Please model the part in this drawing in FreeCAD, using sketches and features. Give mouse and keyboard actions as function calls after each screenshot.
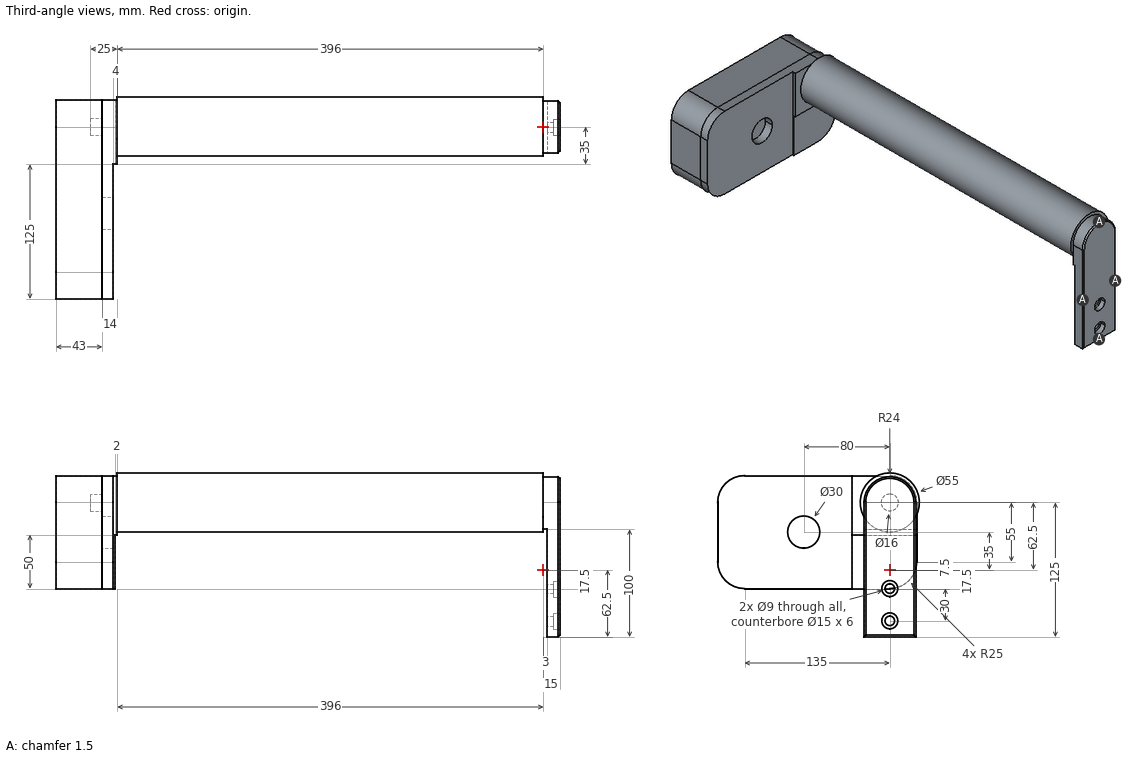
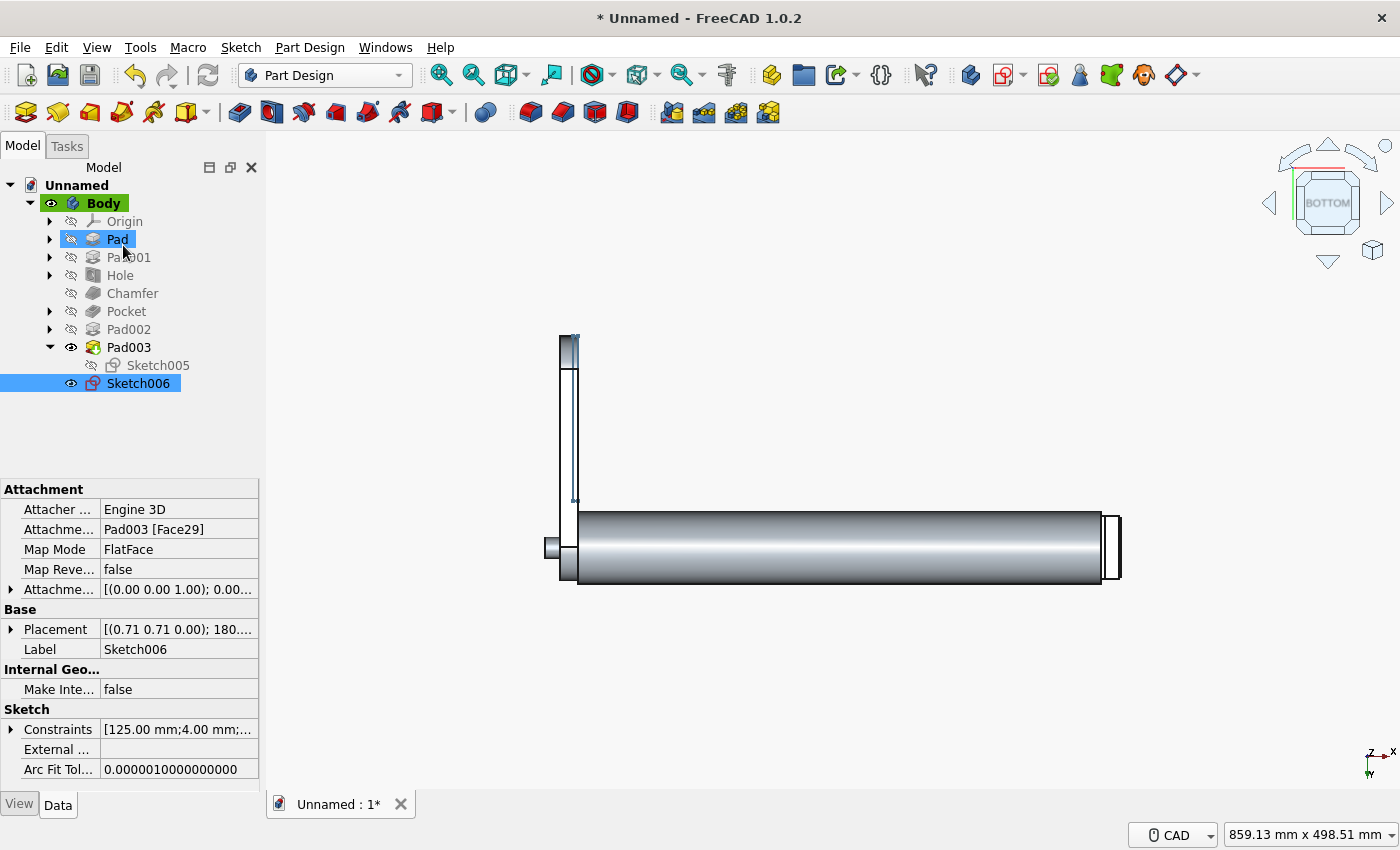
click(240, 112)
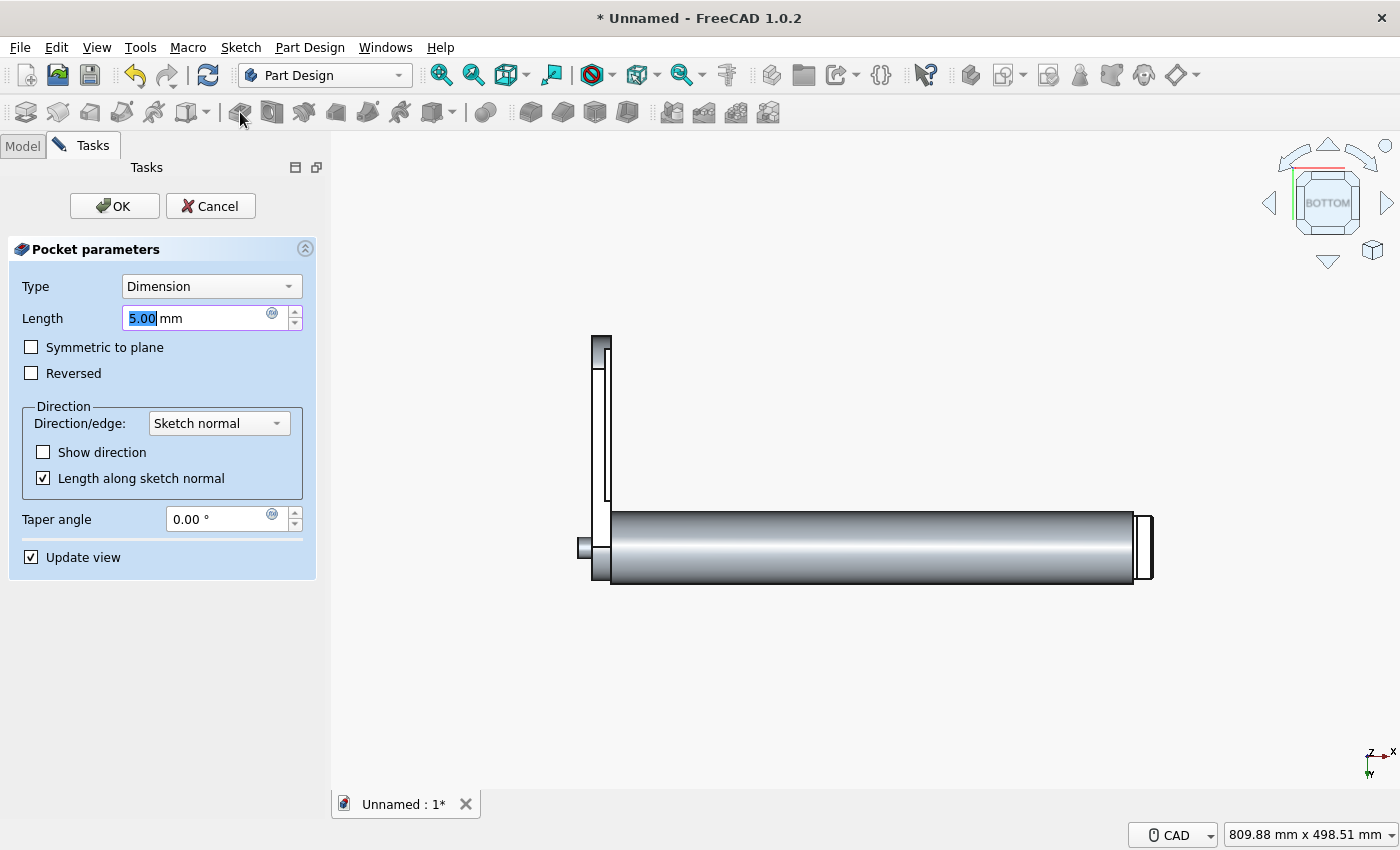
click(212, 286)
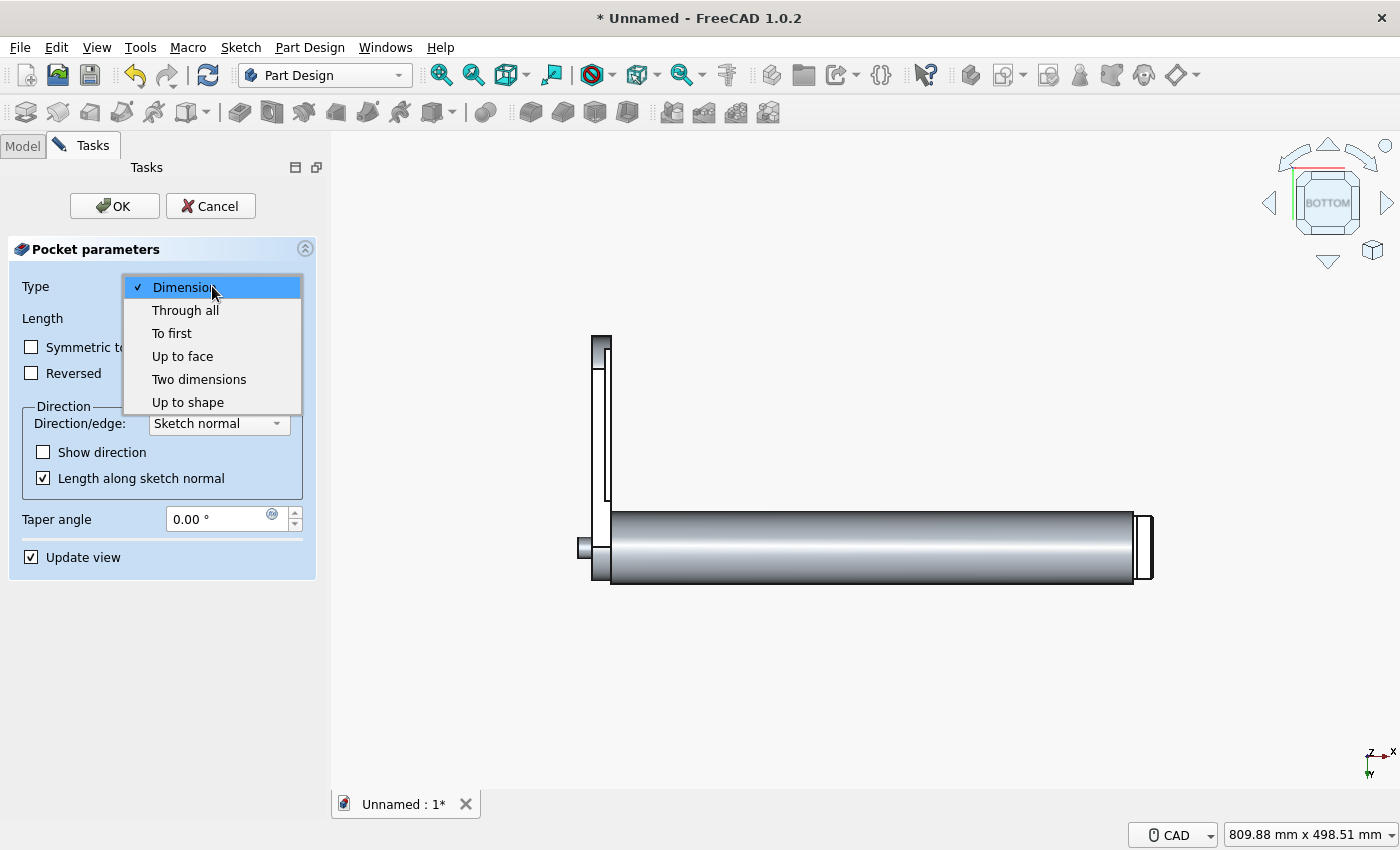
click(212, 310)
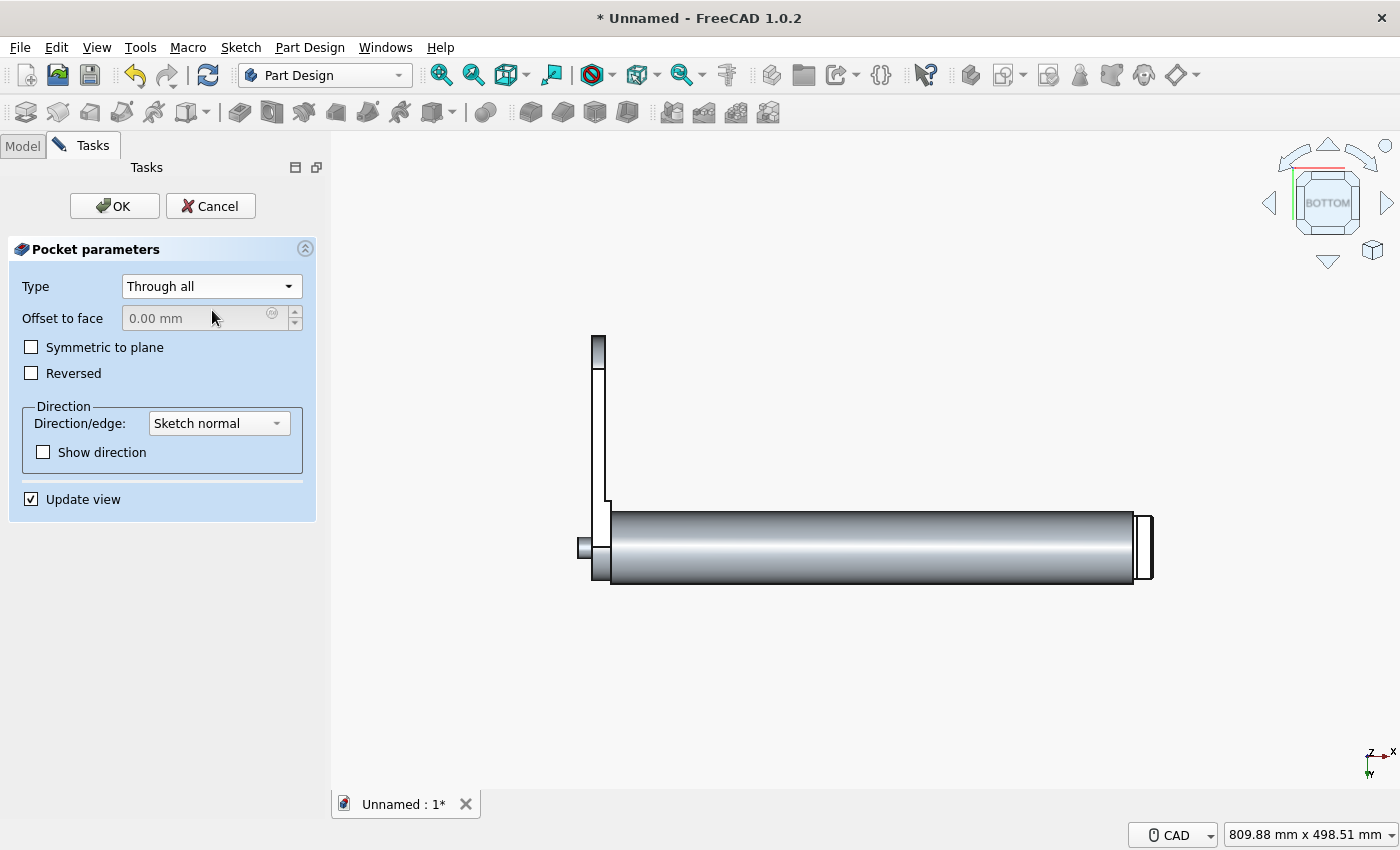
click(115, 206)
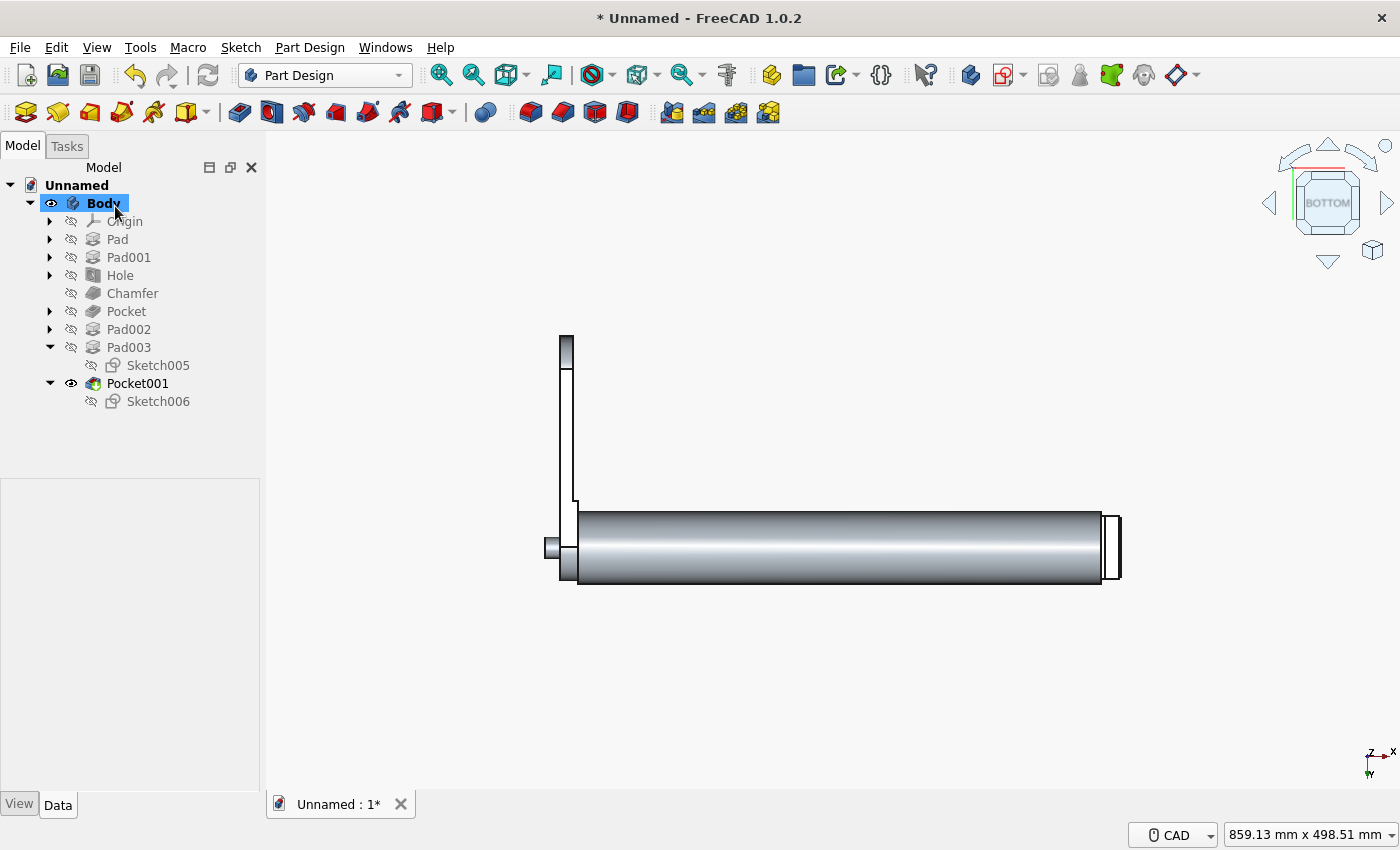
key(0)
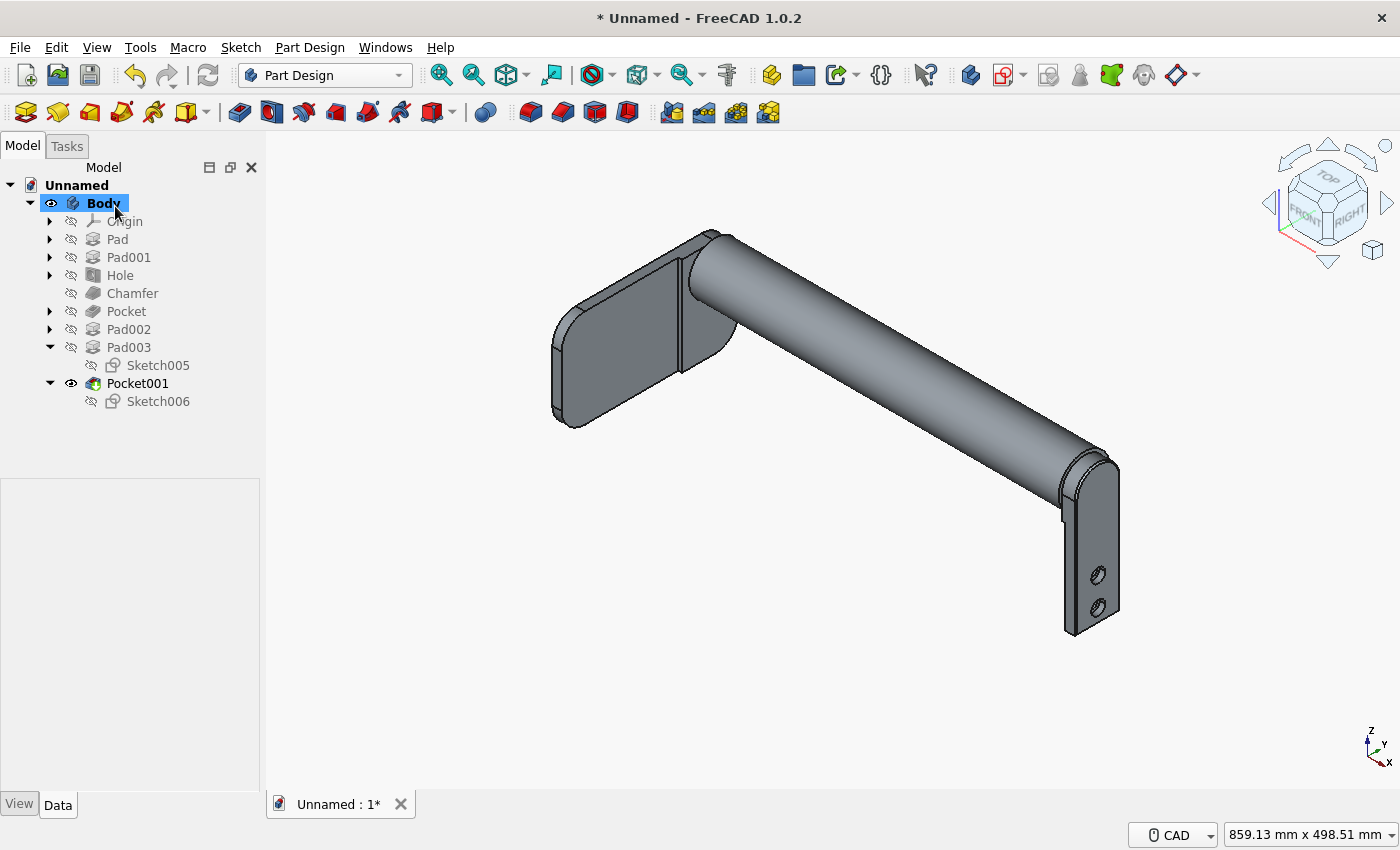
click(620, 347)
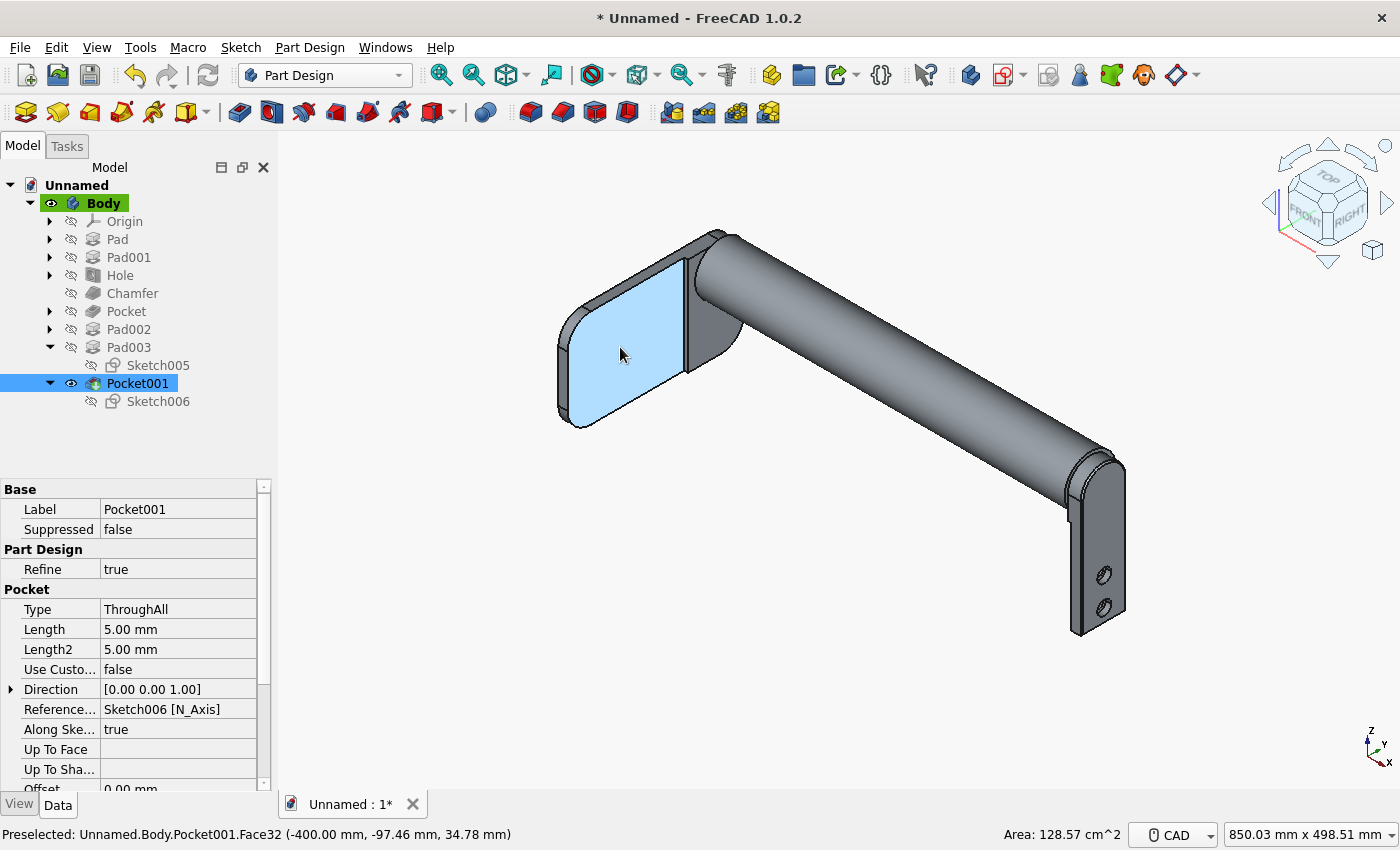
click(1004, 76)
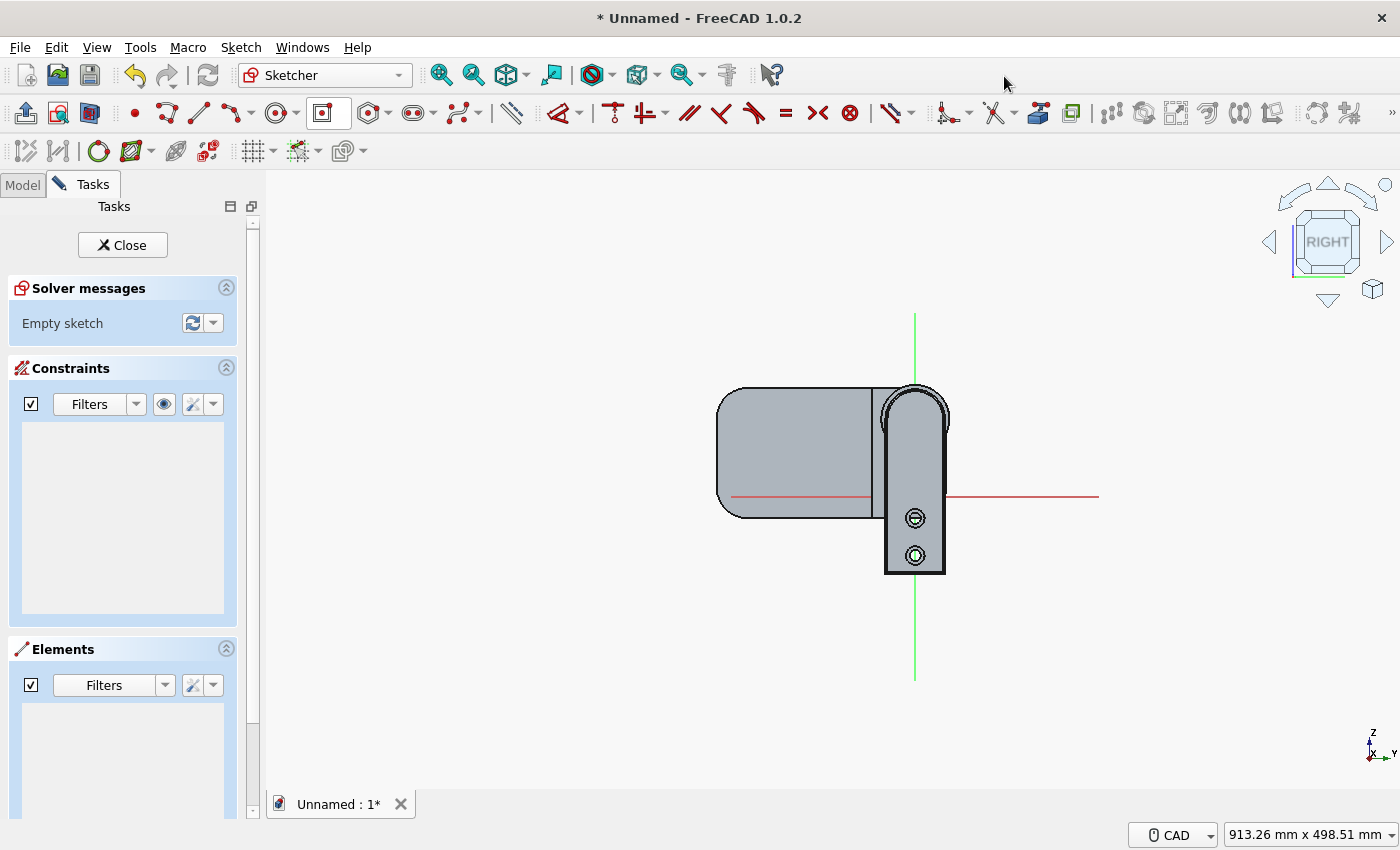
key(q)
key(s)